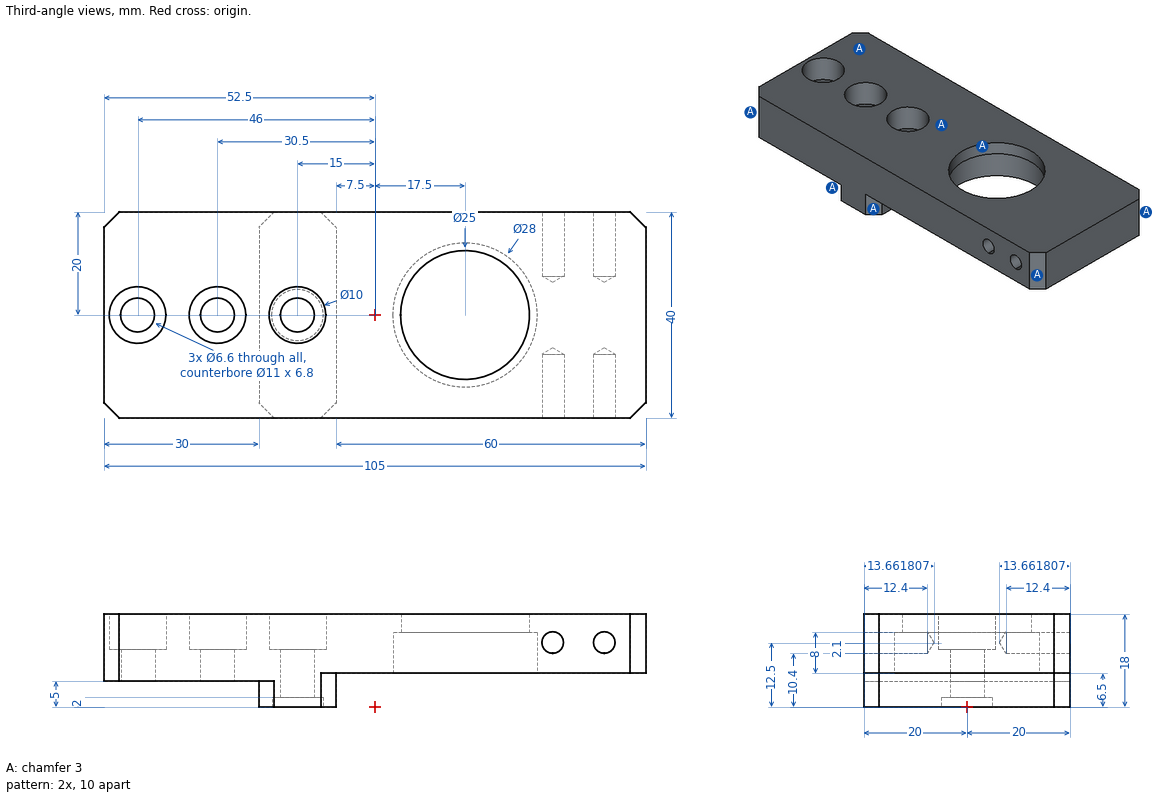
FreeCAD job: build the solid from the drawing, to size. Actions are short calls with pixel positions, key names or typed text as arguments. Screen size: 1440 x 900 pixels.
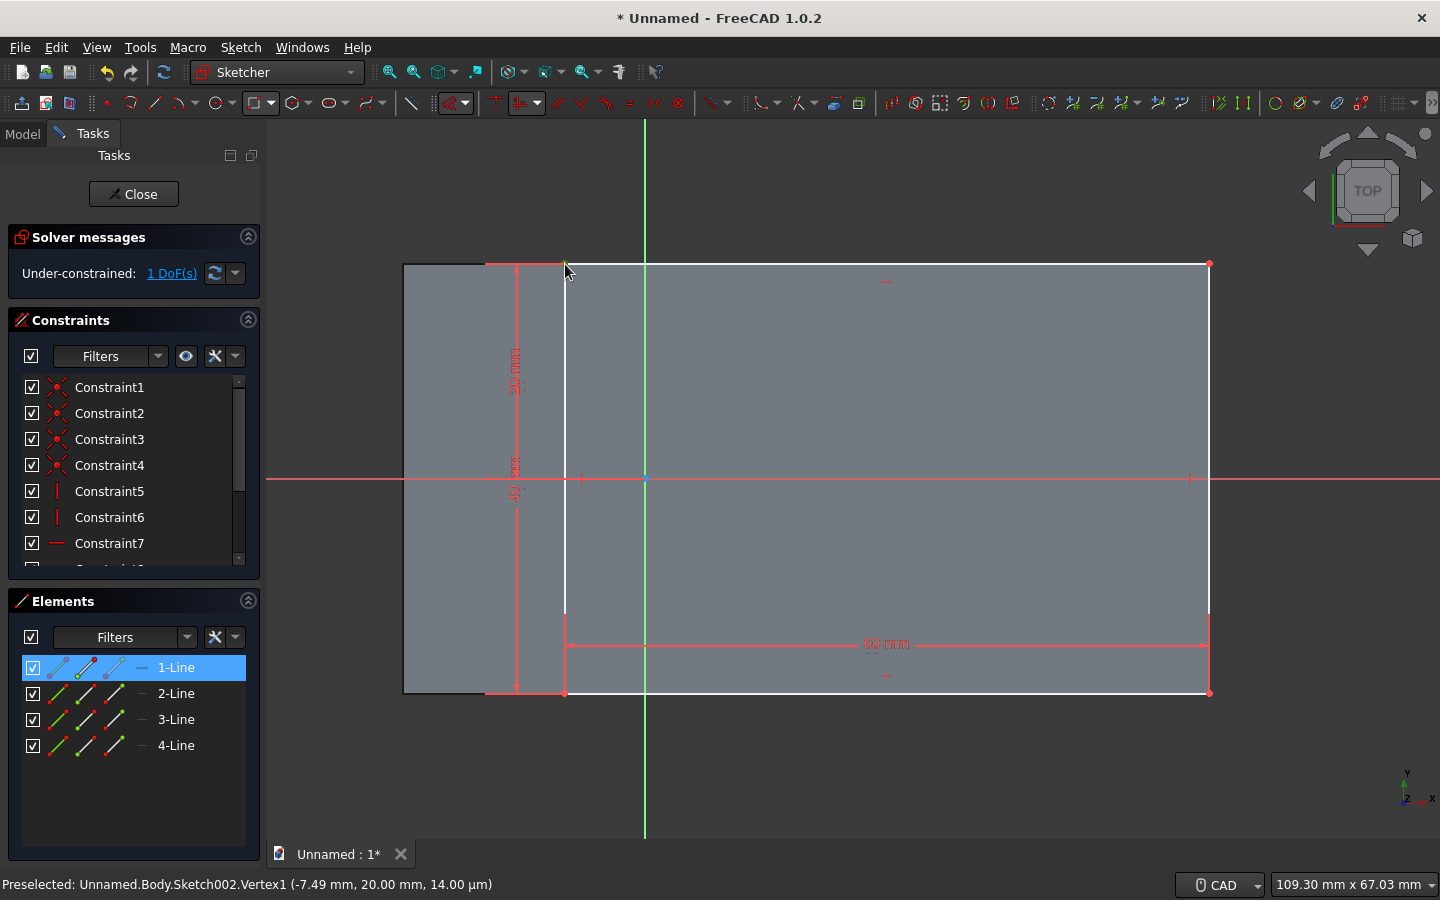
key(l)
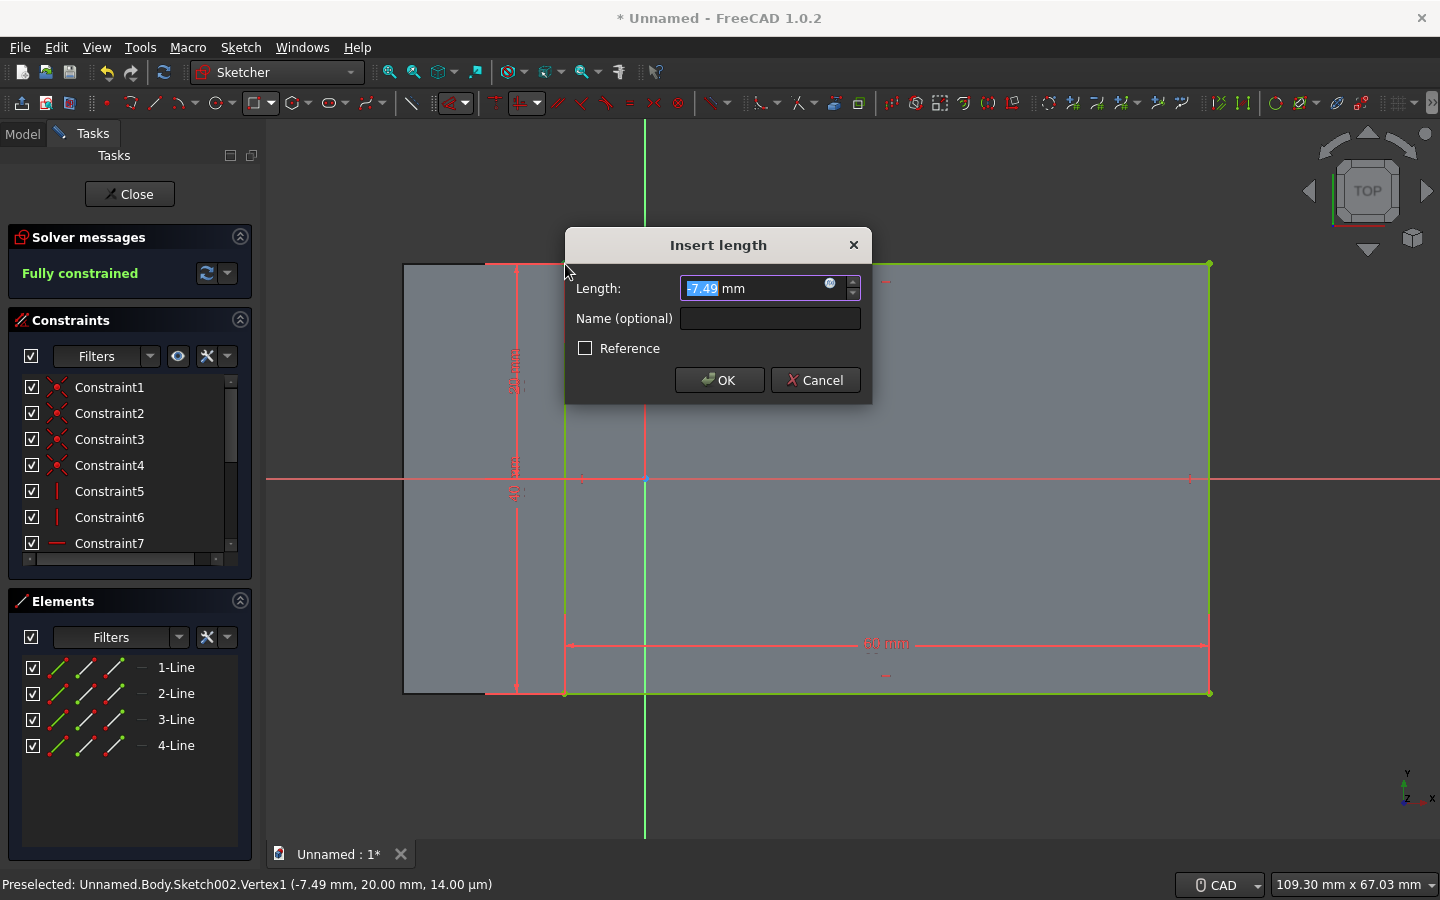
text(-7.5)
key(Return)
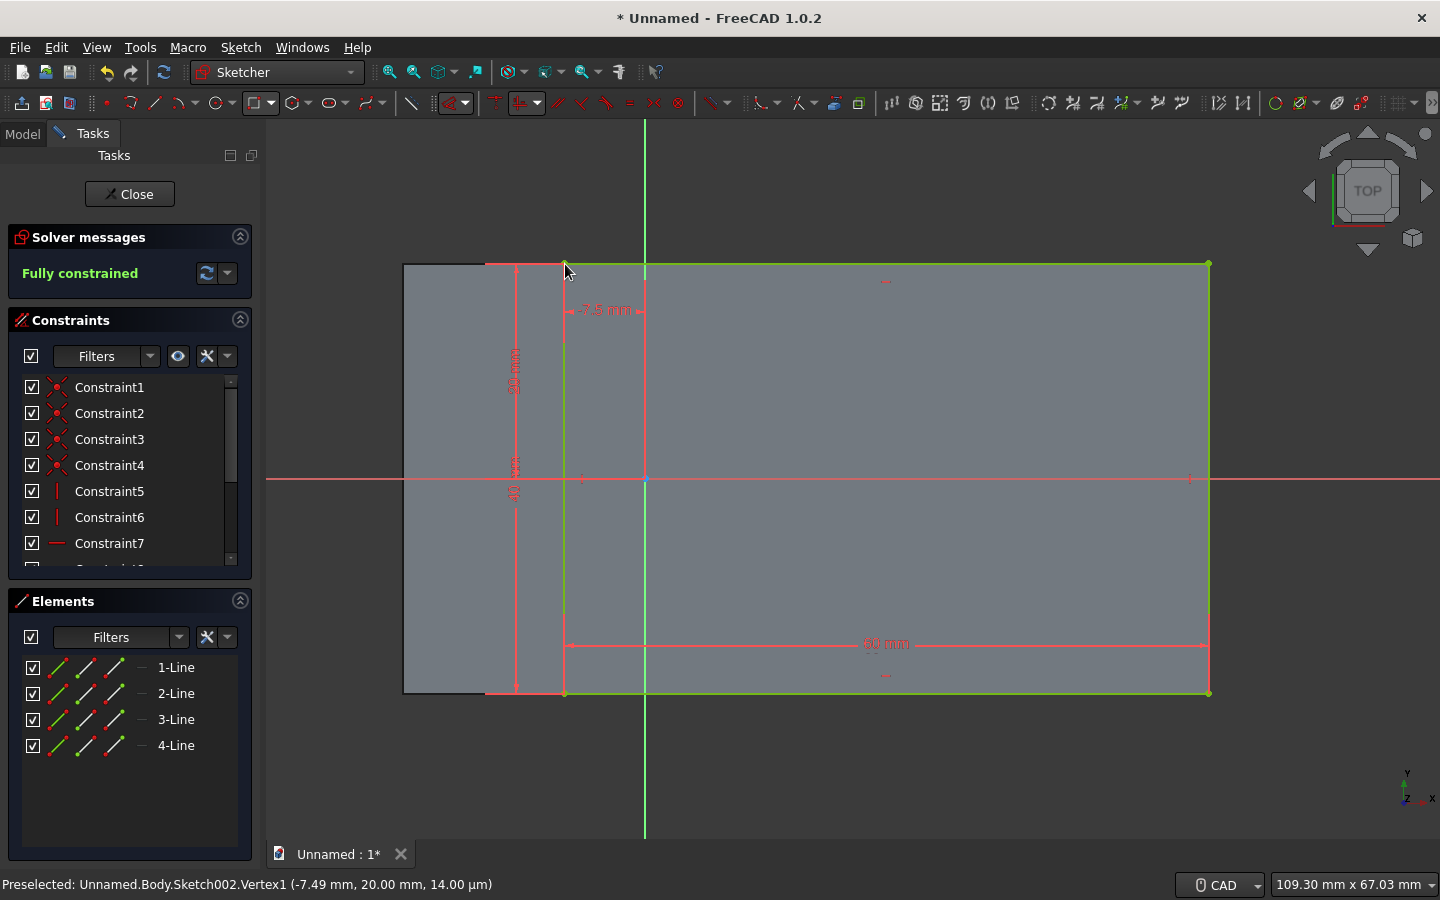
click(130, 194)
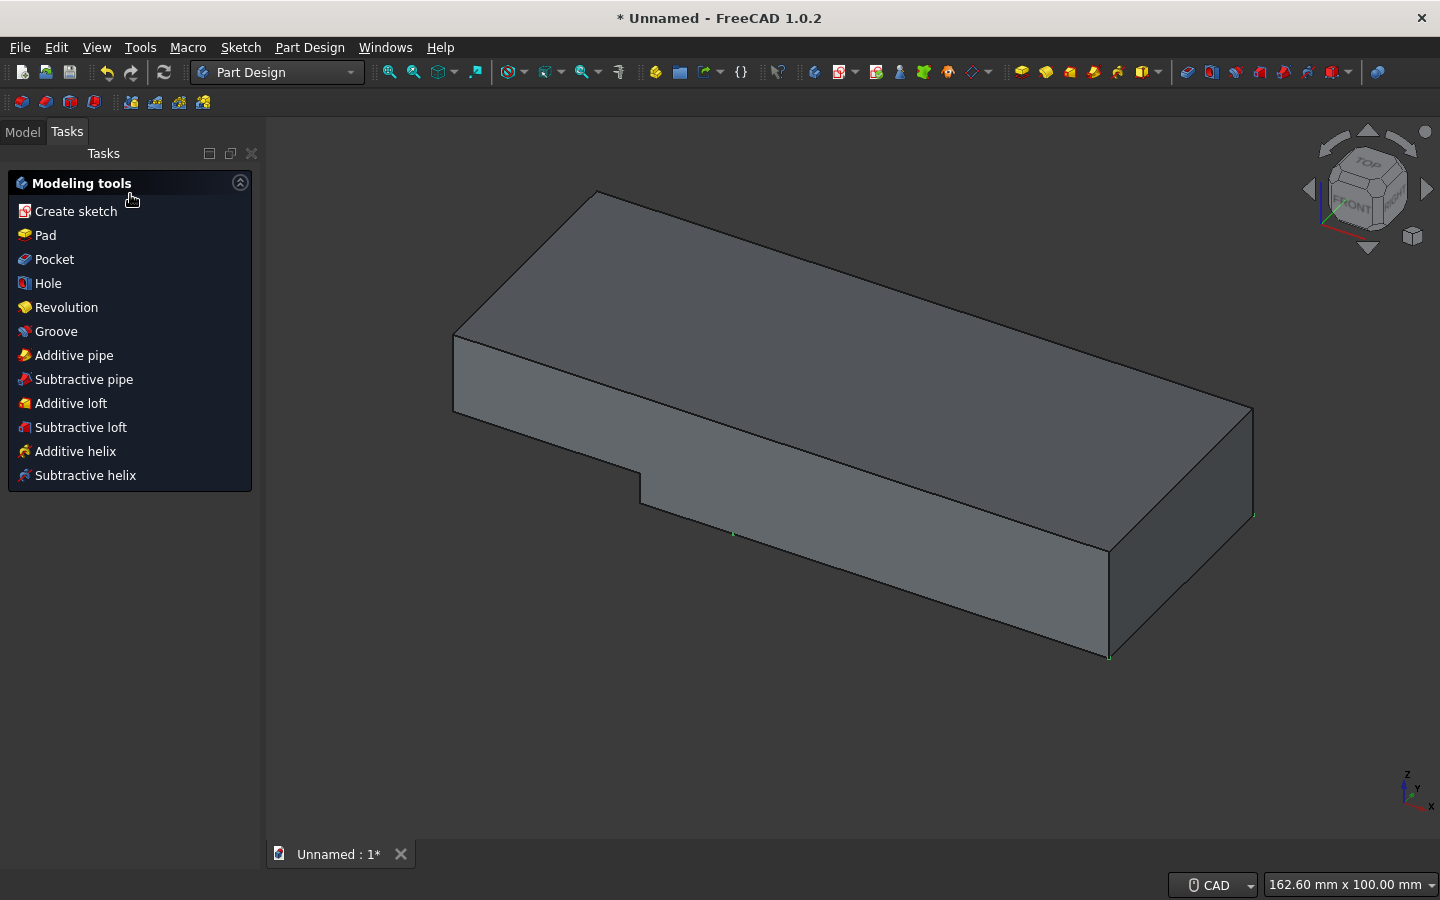
click(1188, 72)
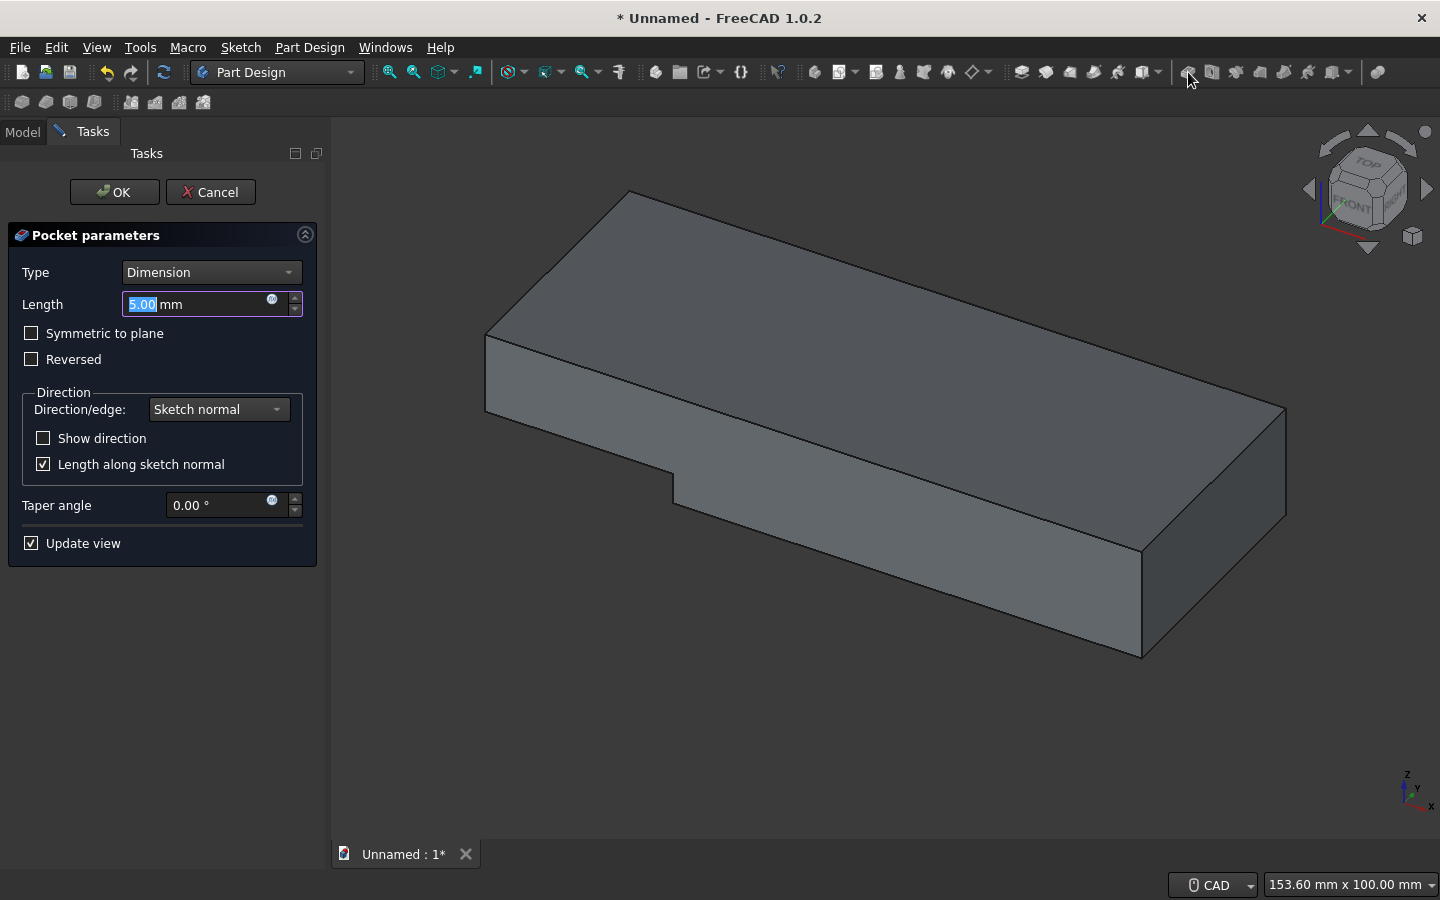
text(6.5)
key(Tab)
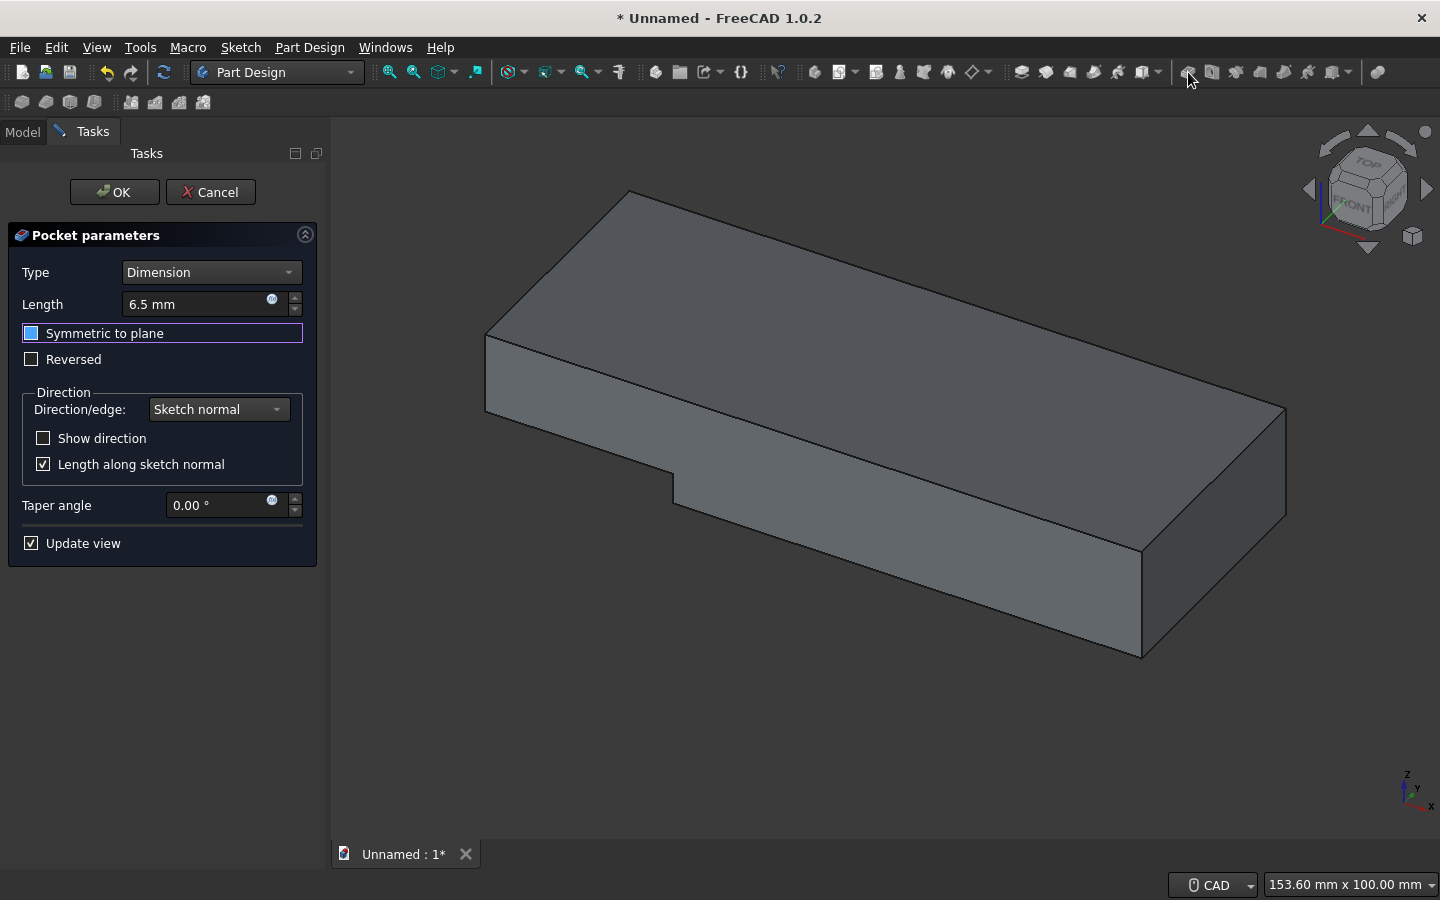
click(30, 359)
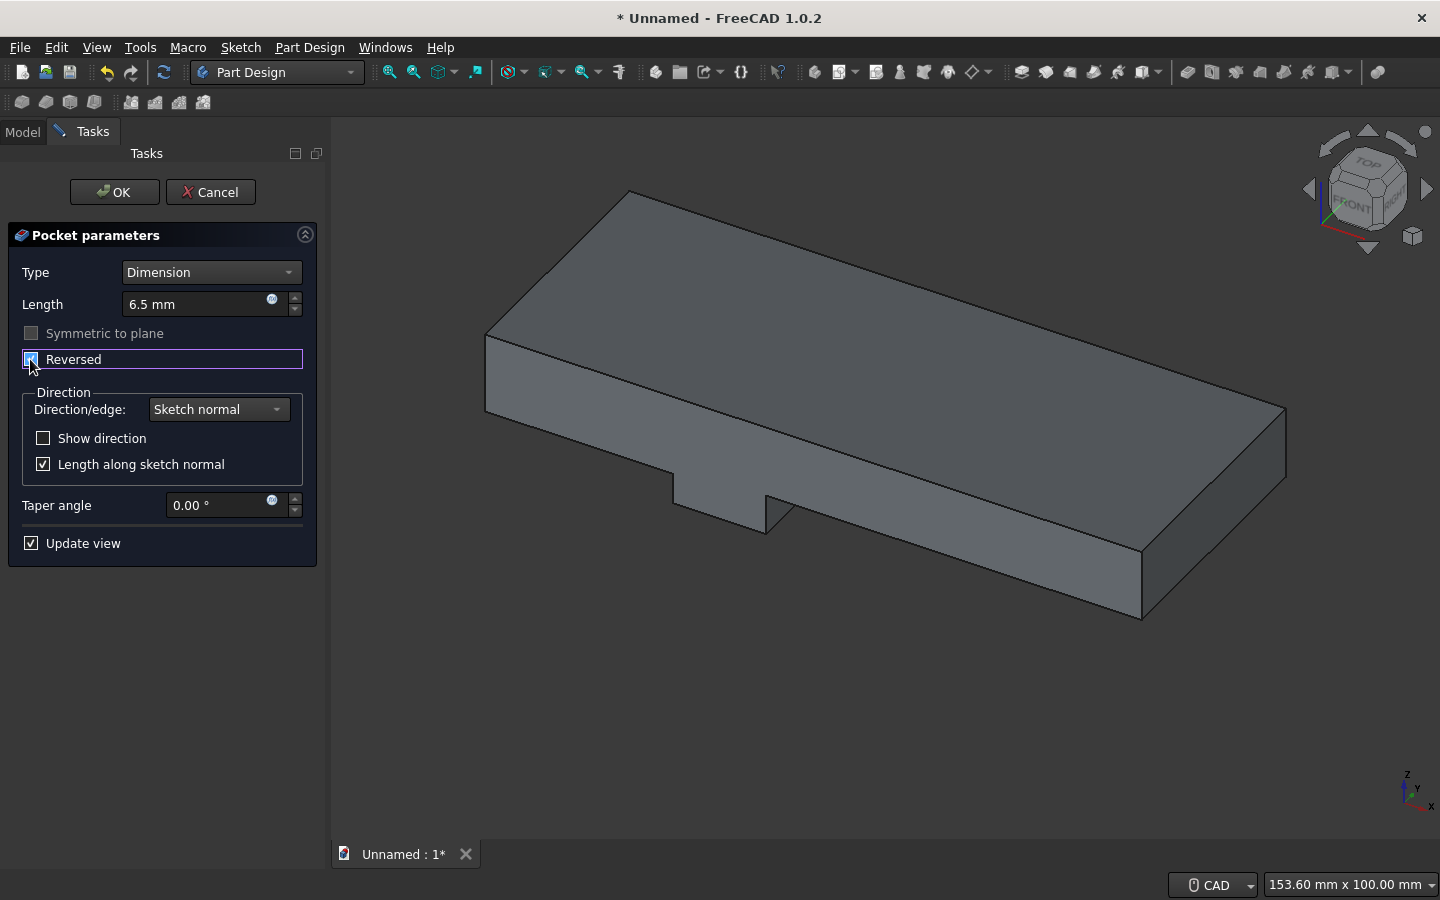
click(115, 192)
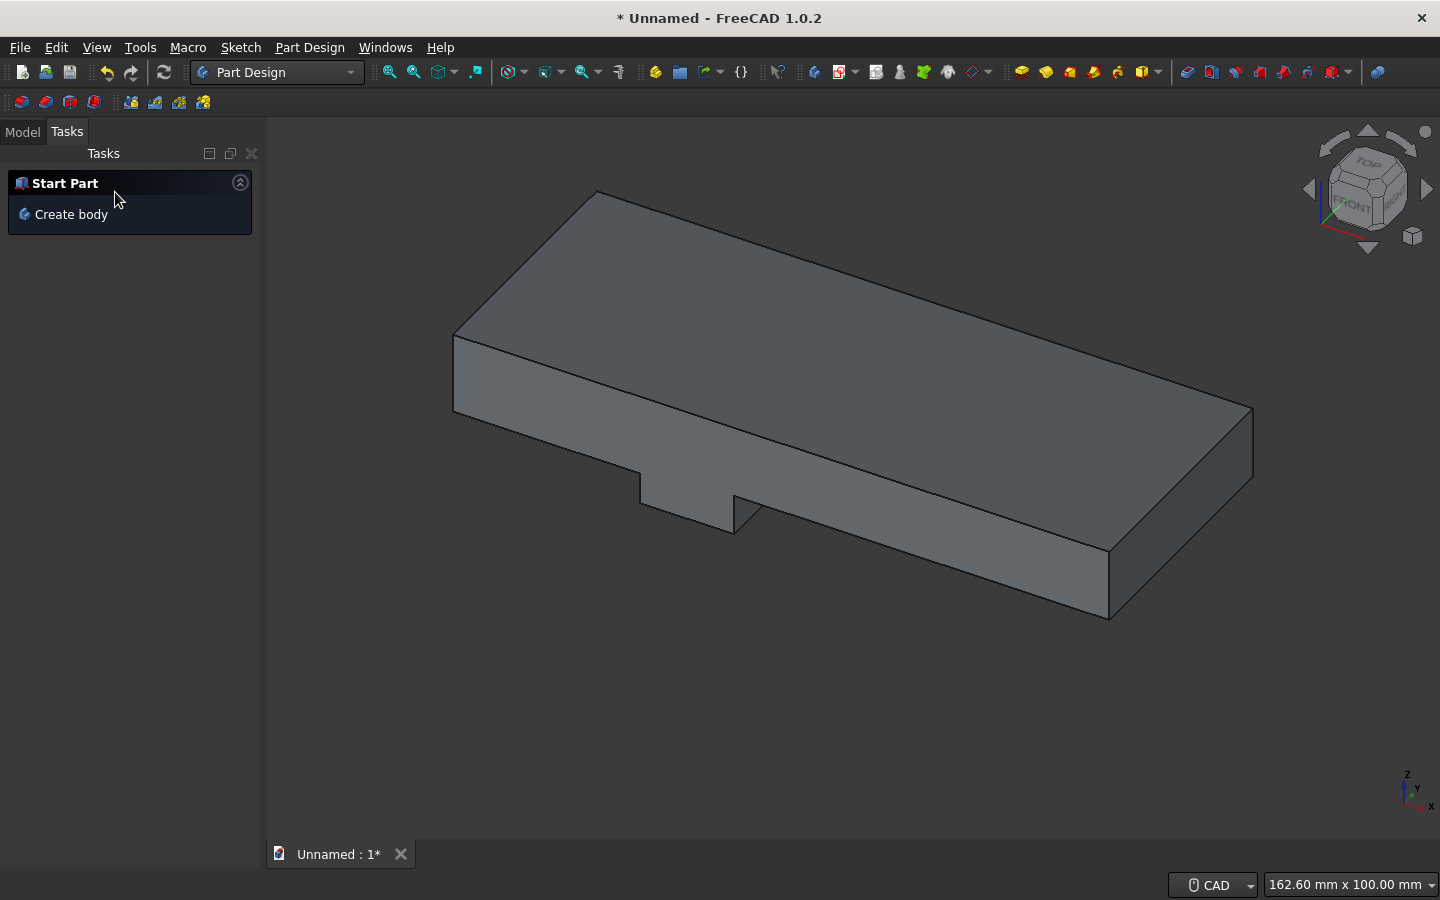
click(1041, 433)